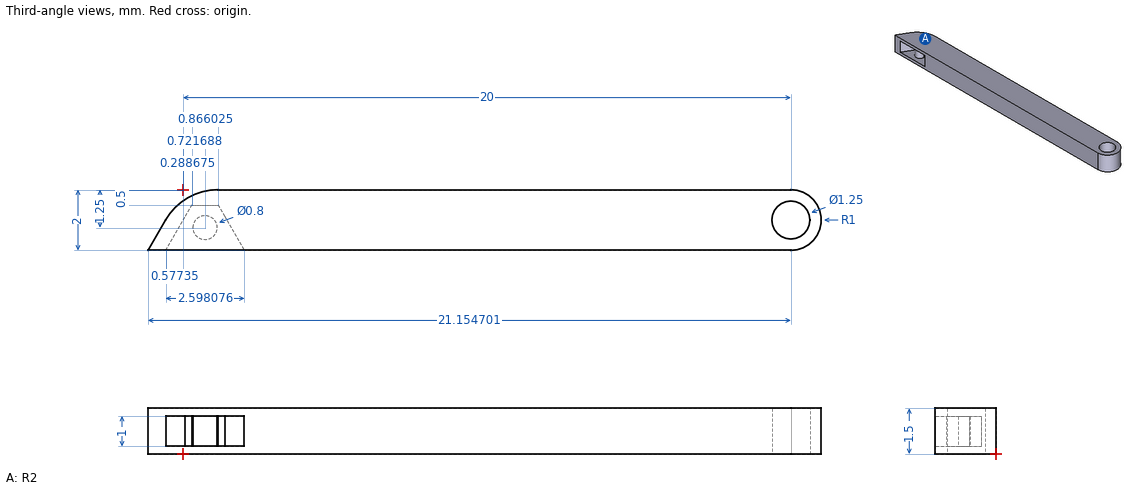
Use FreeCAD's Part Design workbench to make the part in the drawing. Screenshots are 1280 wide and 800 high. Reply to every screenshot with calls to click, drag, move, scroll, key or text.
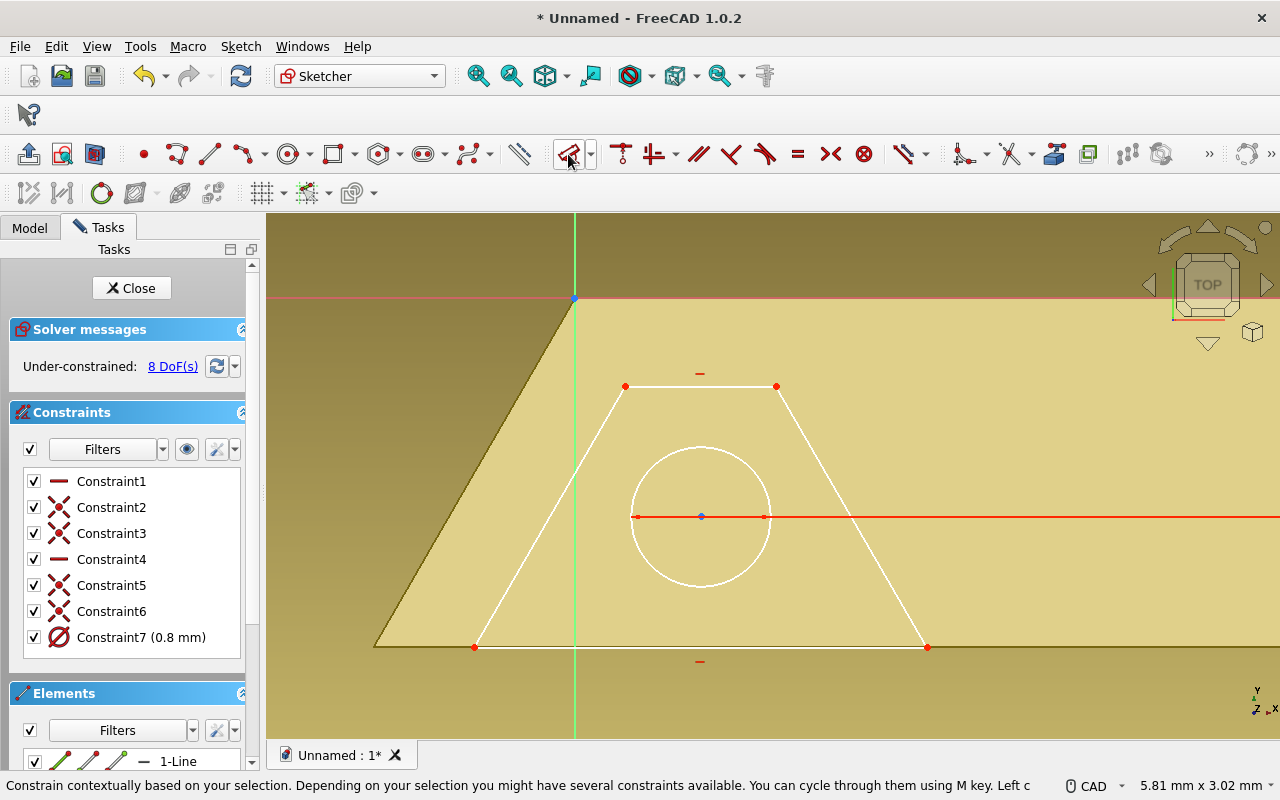
click(927, 648)
click(961, 473)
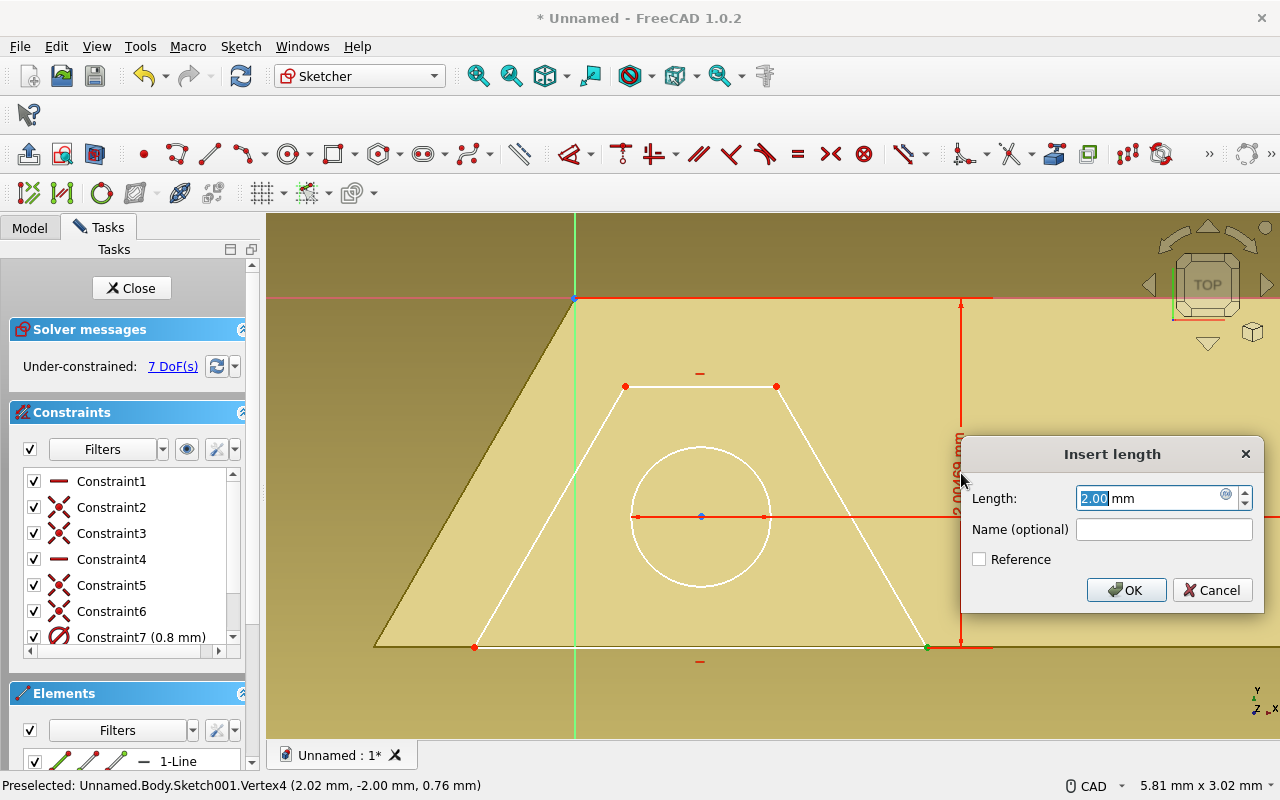
text(2)
key(Return)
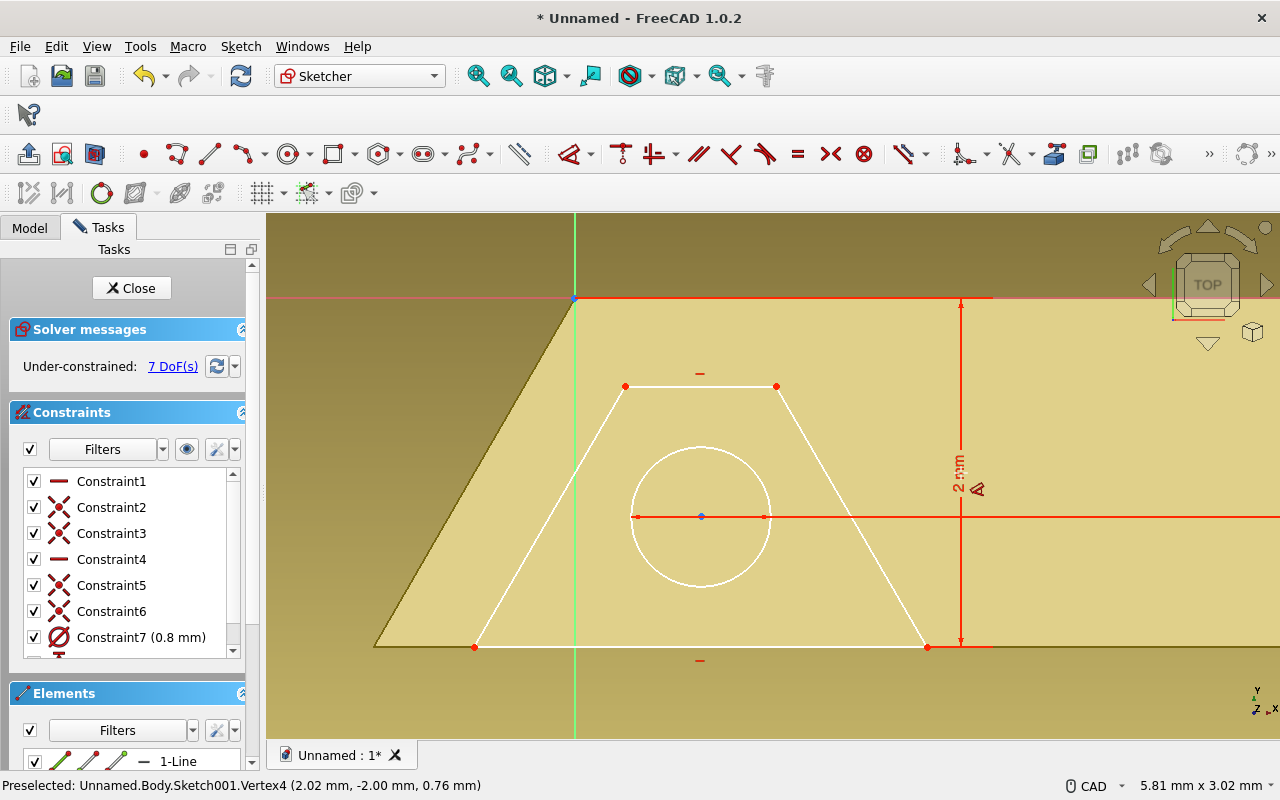
click(625, 387)
click(541, 343)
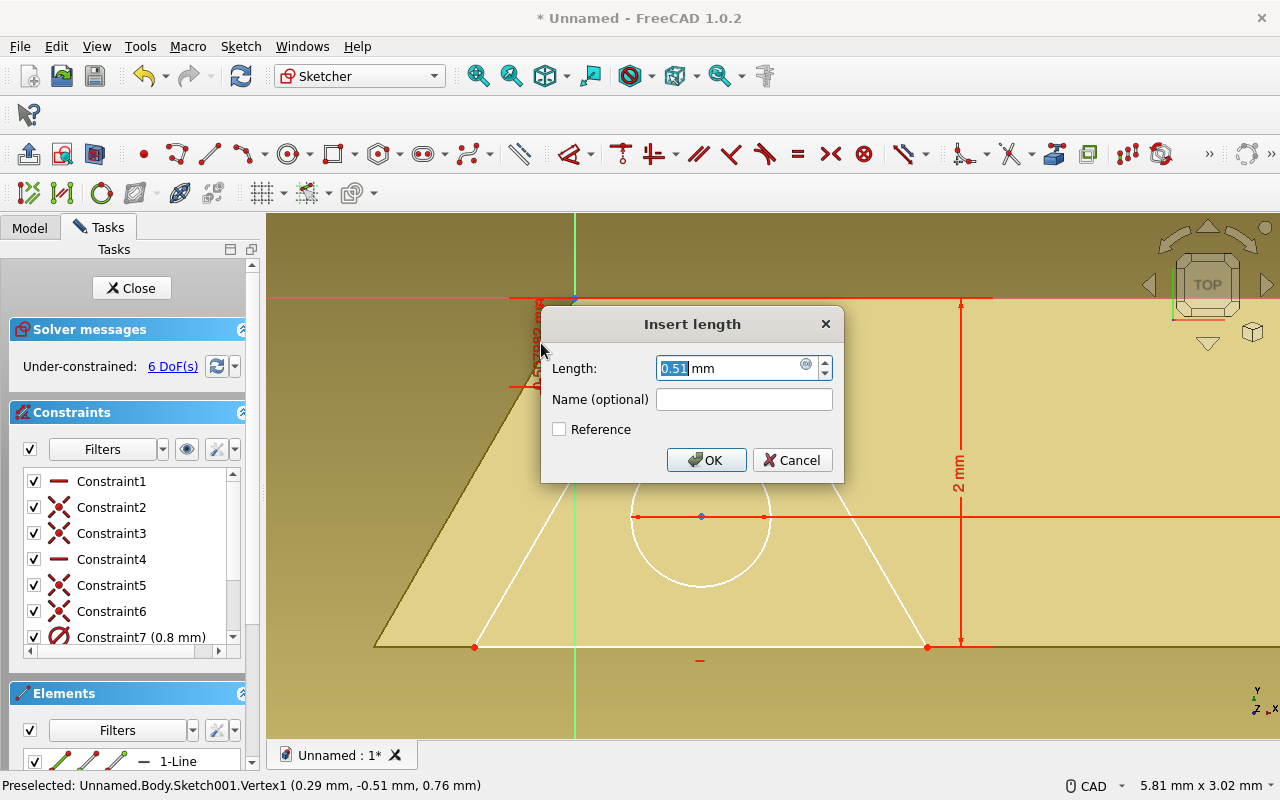
text(0.5)
key(Return)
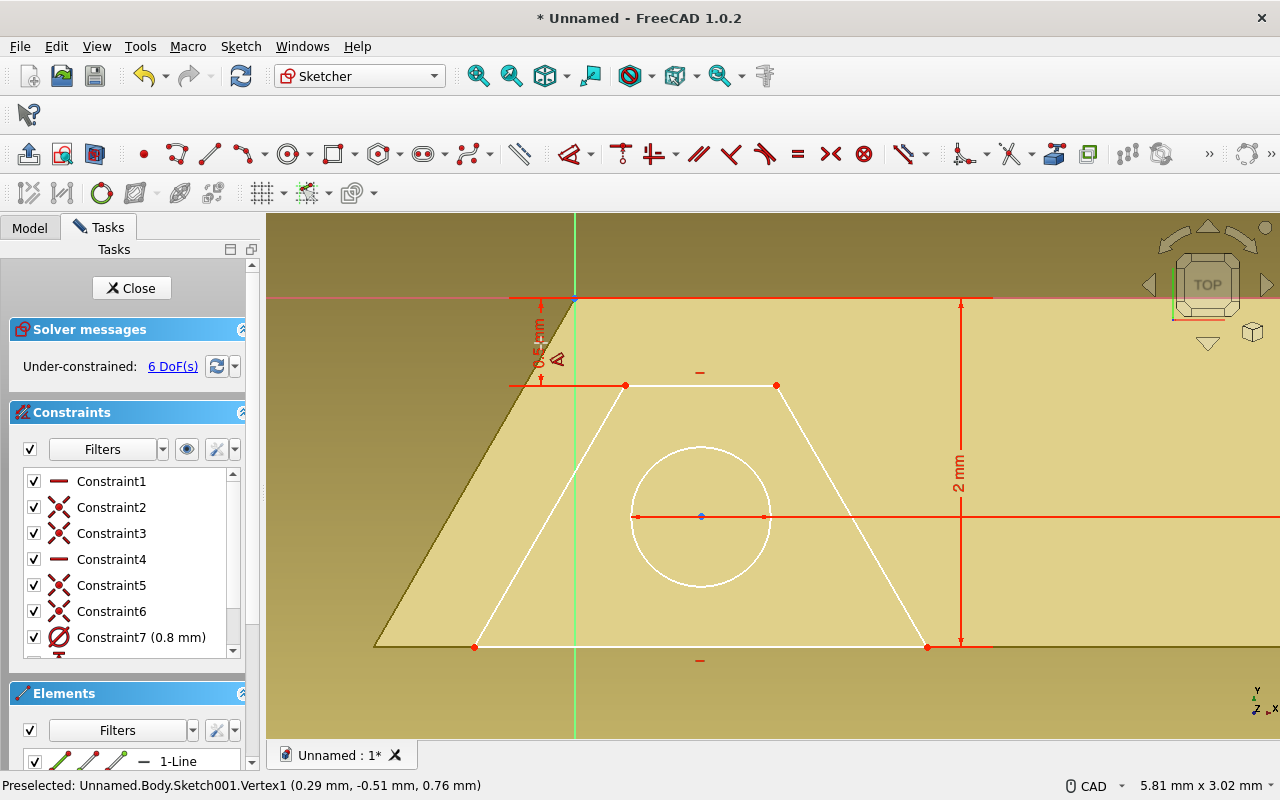
click(701, 517)
click(541, 408)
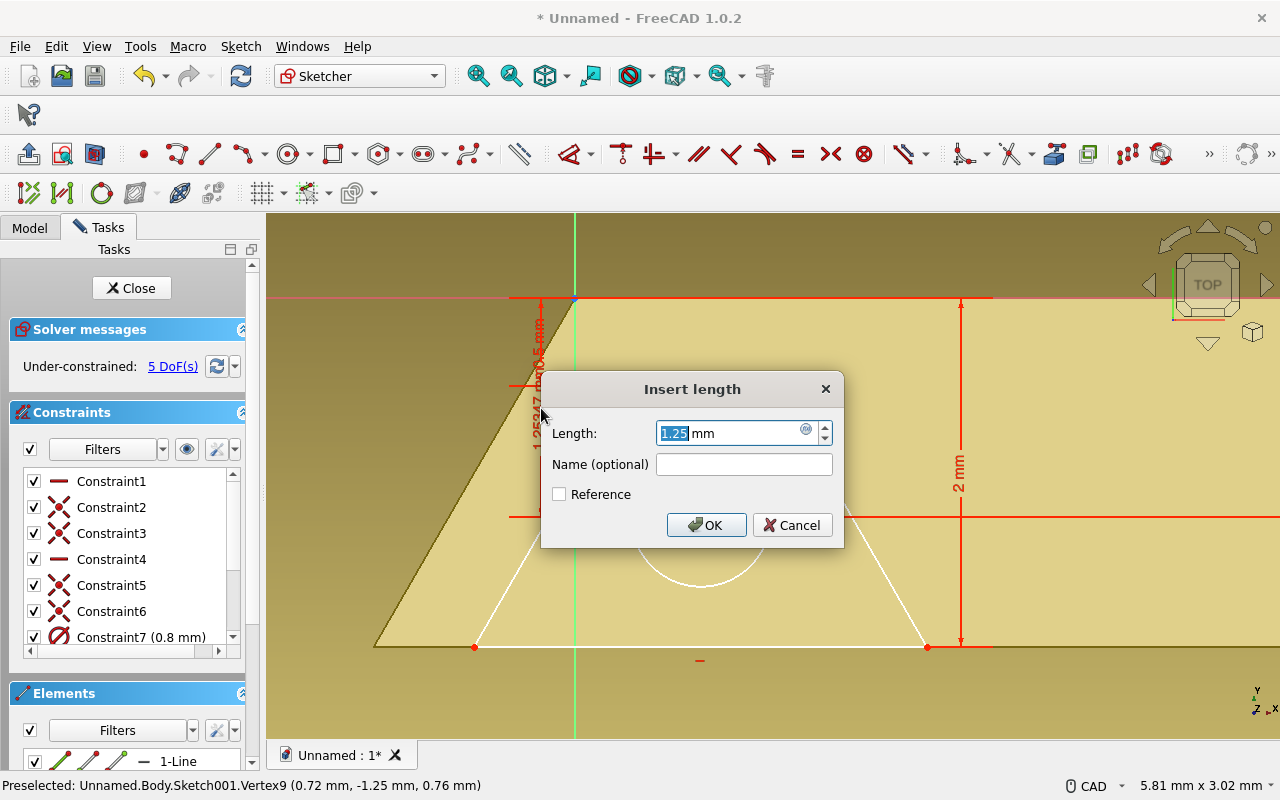
text(1.25)
key(Return)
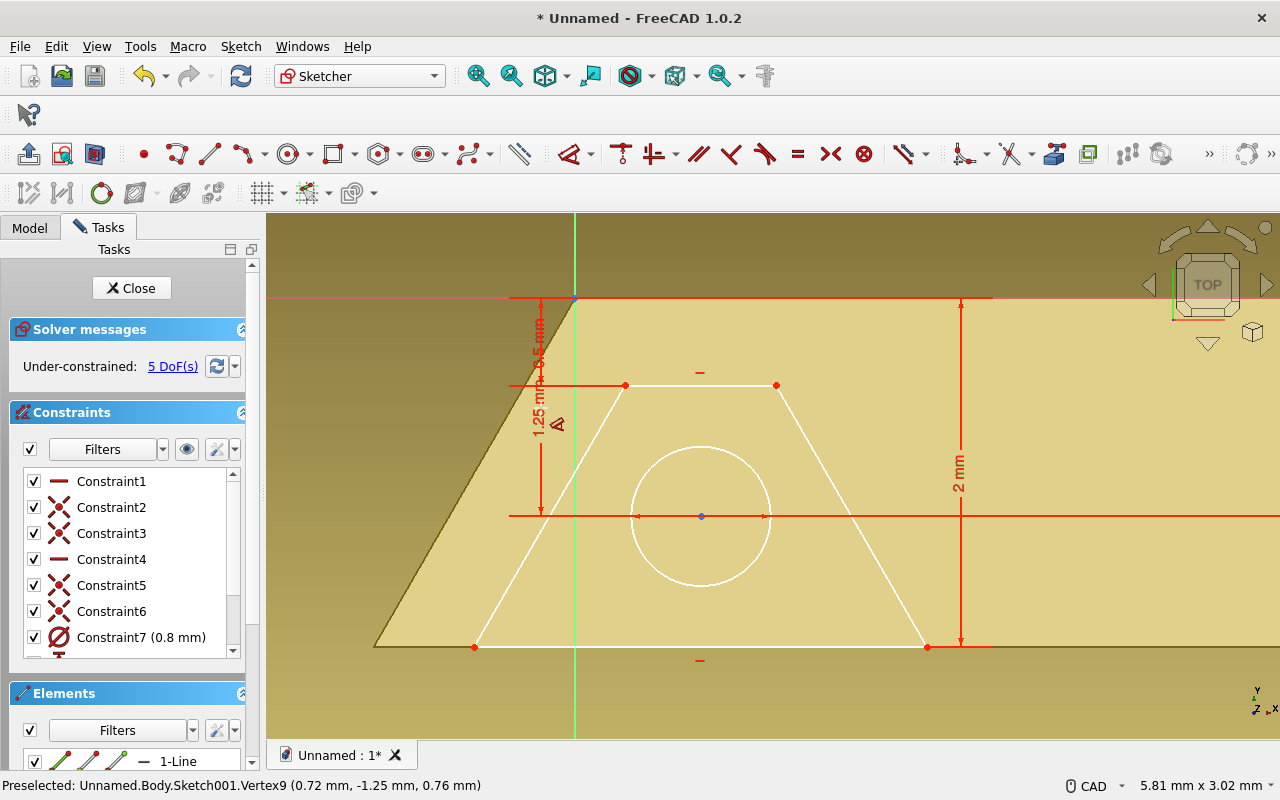
click(670, 386)
click(701, 352)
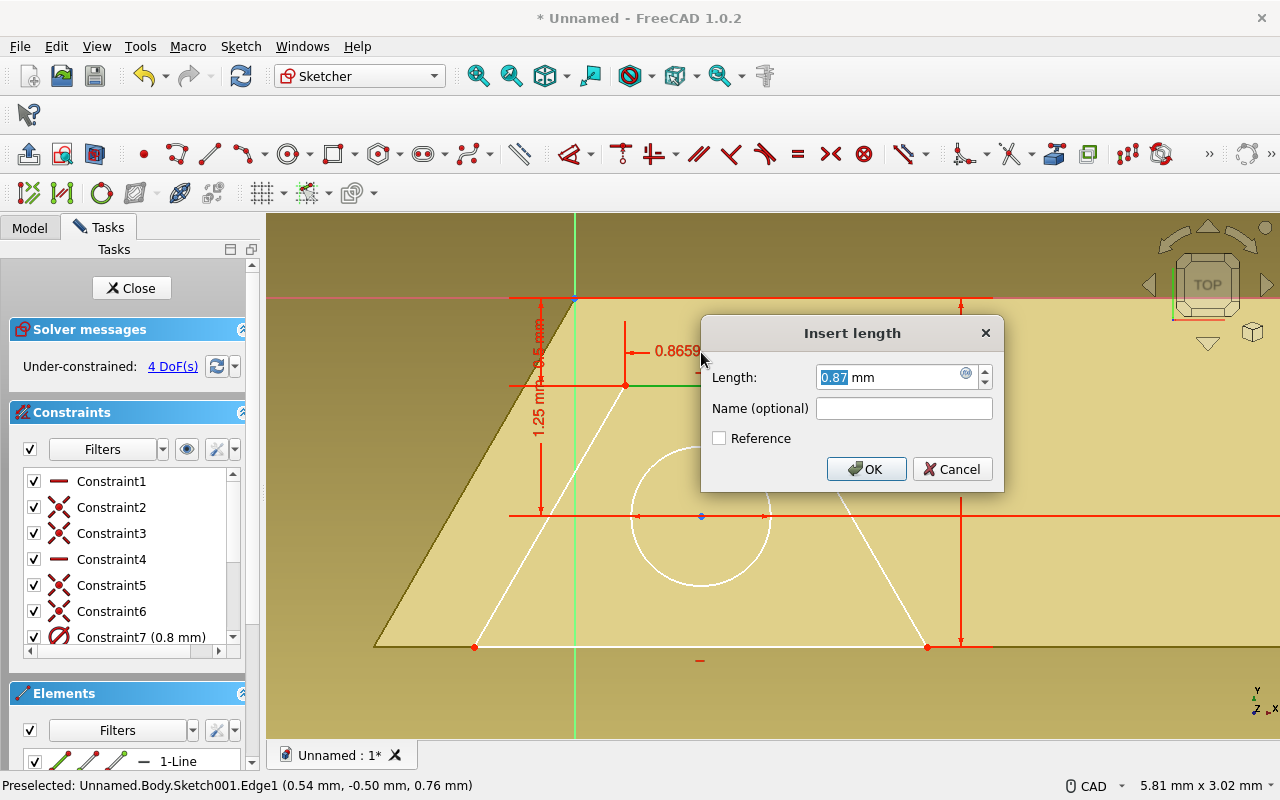
text(0.866025)
key(Return)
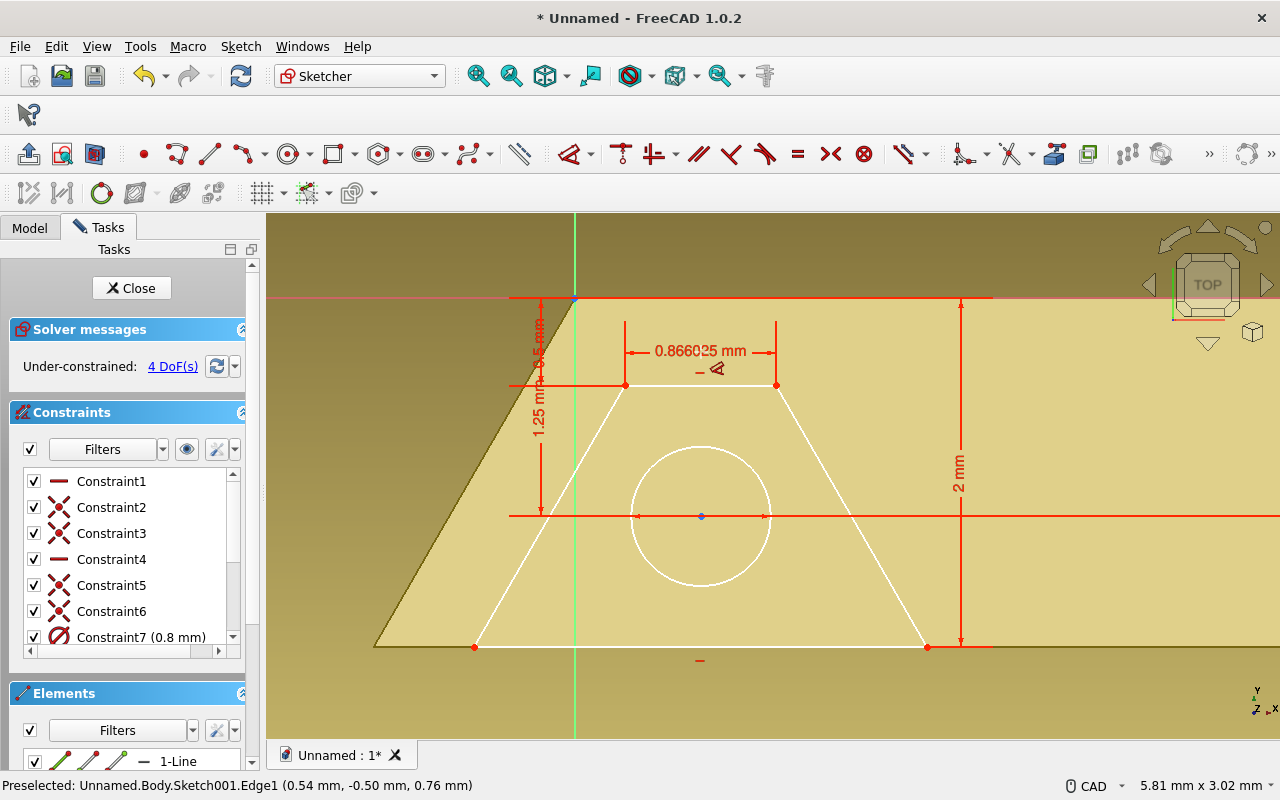
click(791, 647)
click(701, 681)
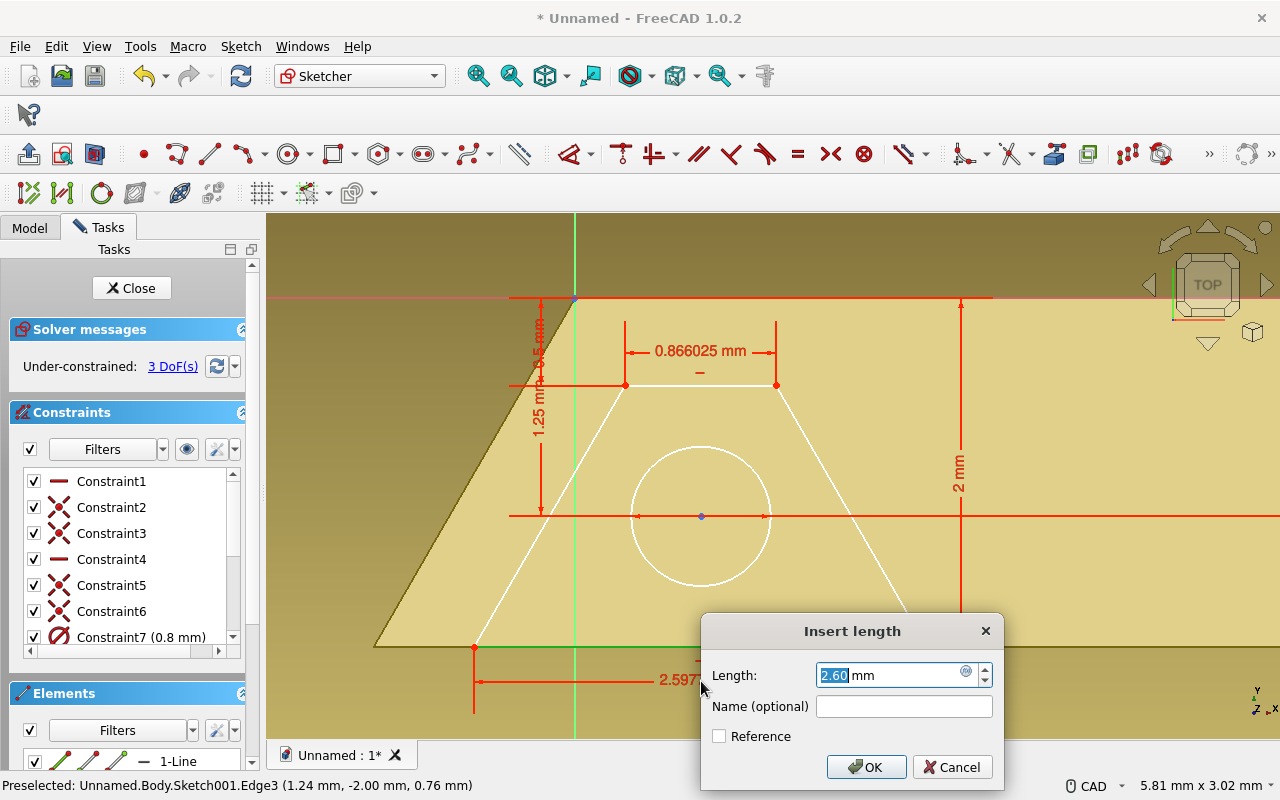
text(2.598076)
key(Return)